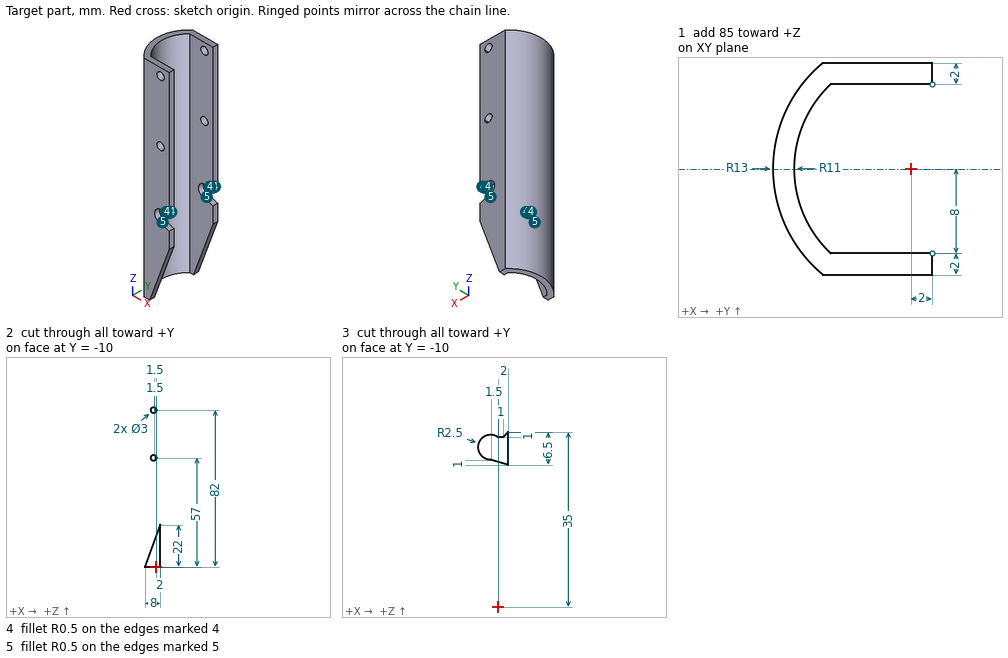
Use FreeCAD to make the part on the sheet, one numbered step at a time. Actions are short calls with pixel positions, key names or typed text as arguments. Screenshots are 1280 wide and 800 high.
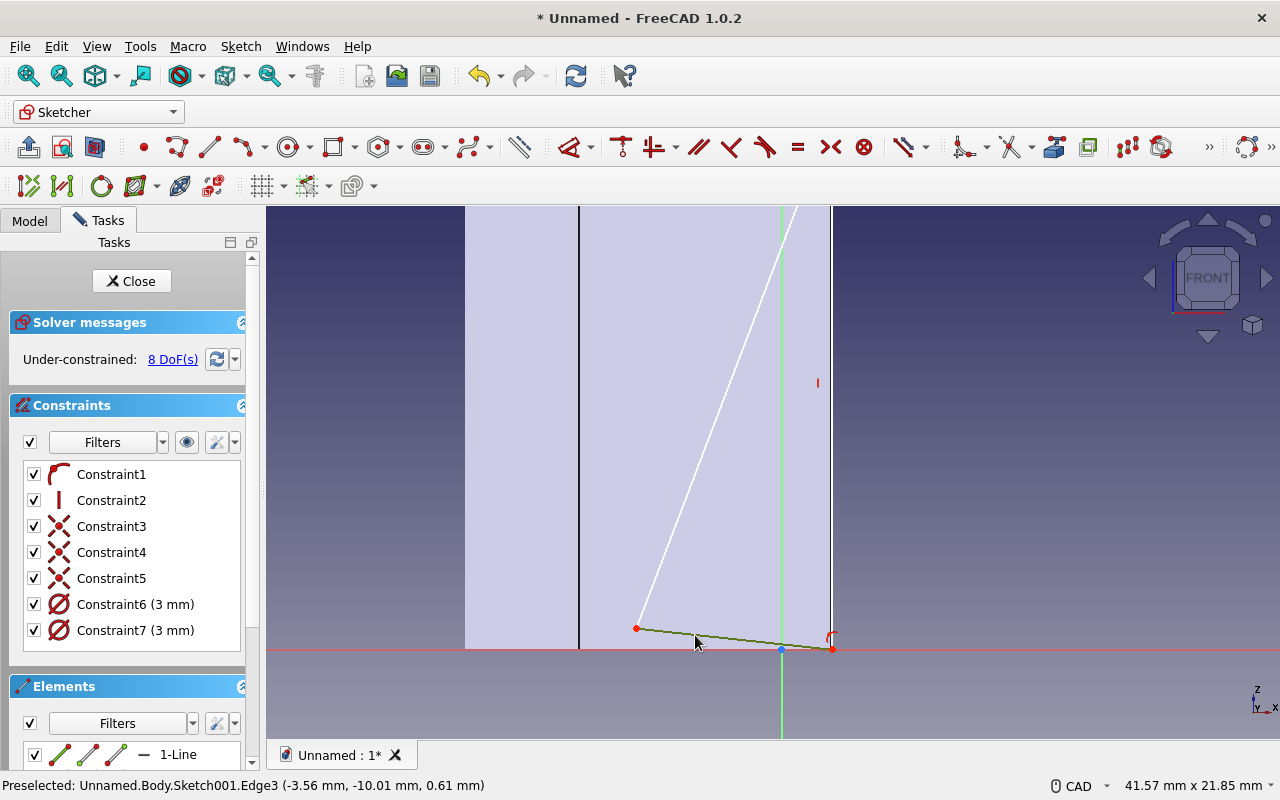
key(h)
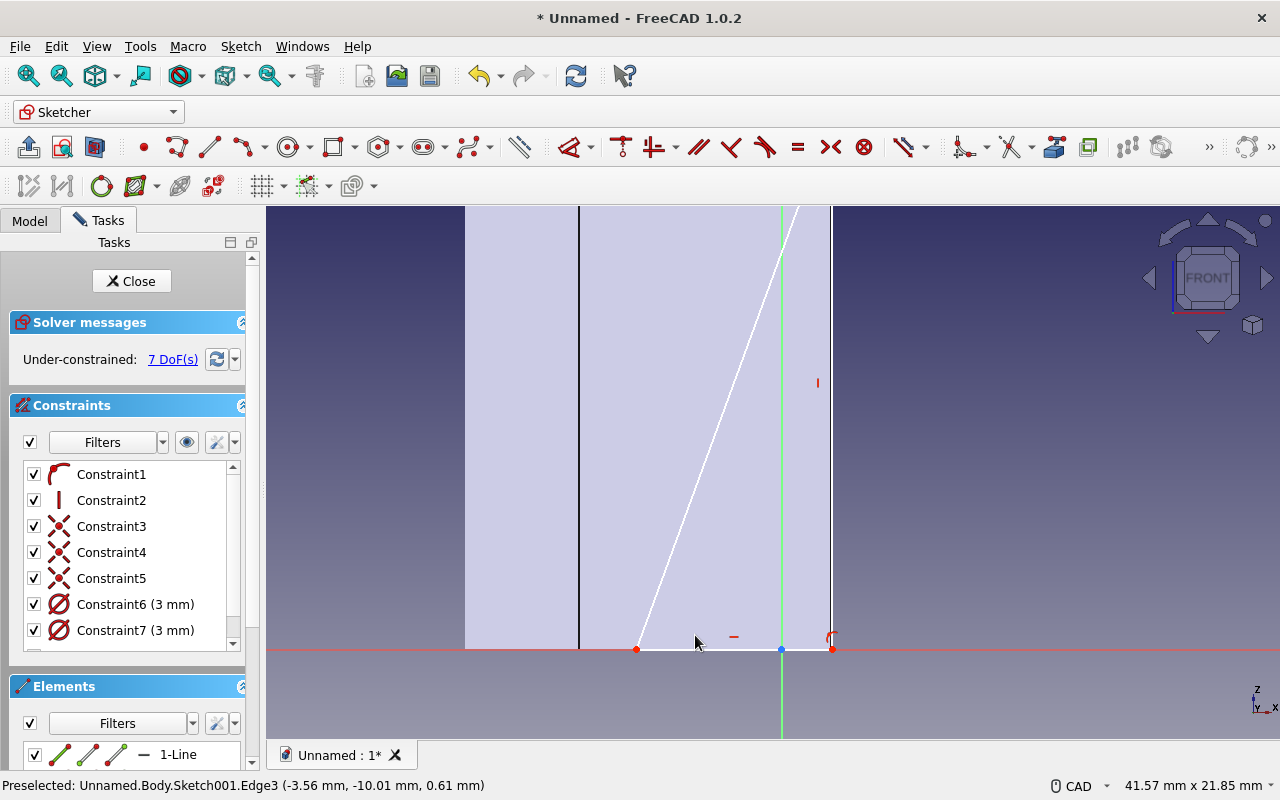
key(d)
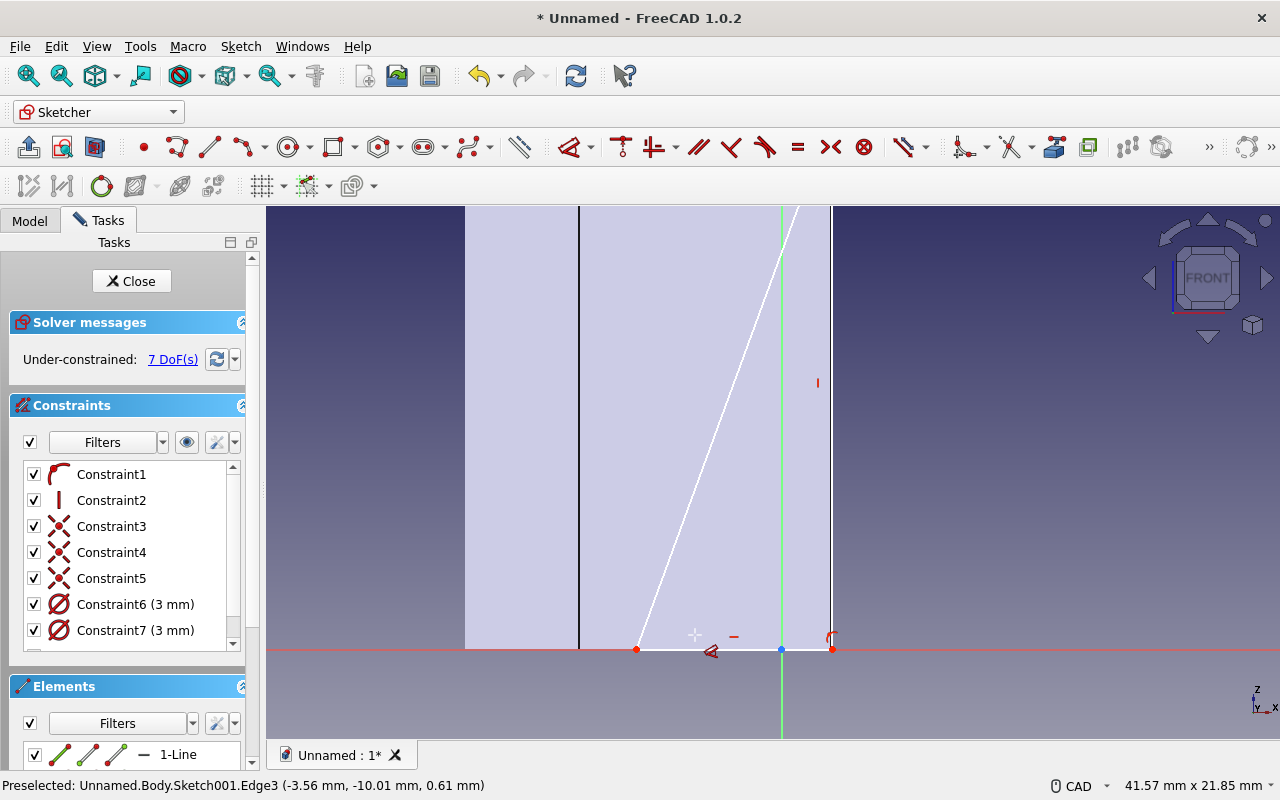
scroll(699, 639, down, 9)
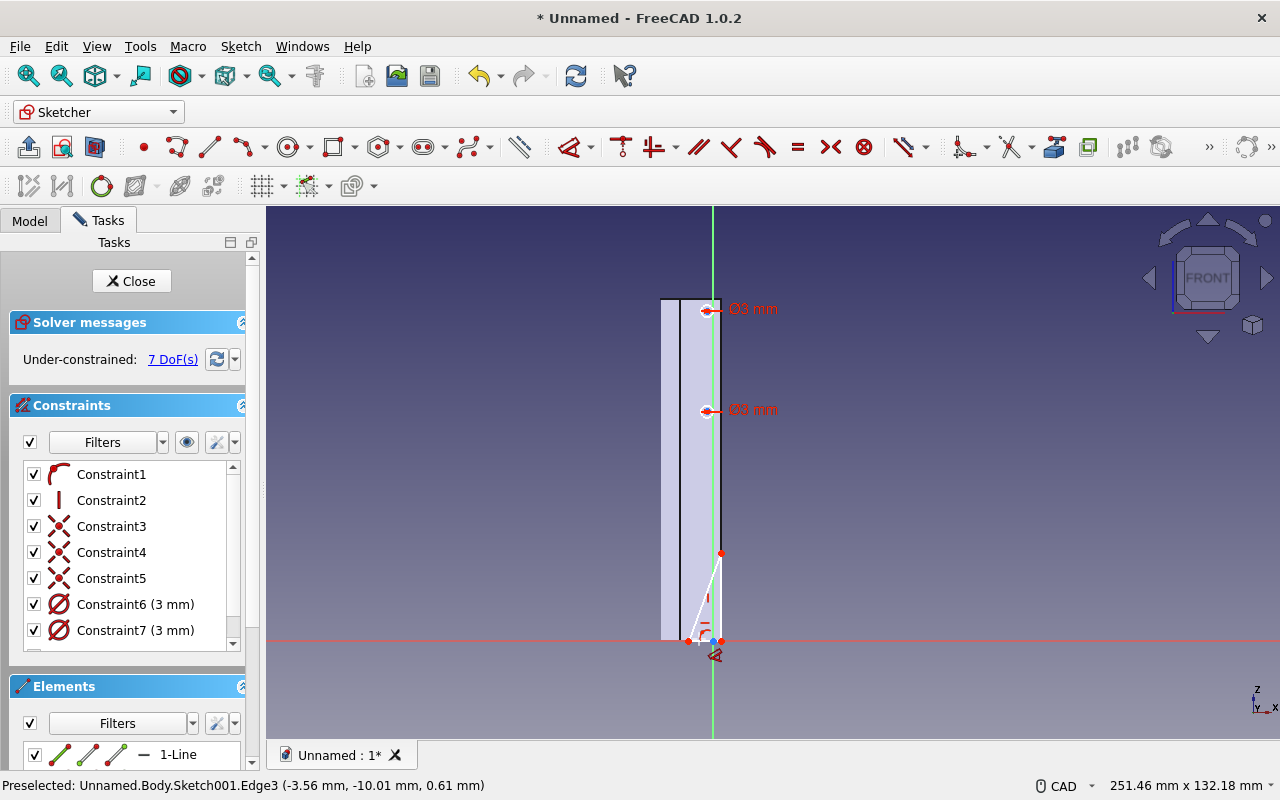
scroll(699, 641, up, 3)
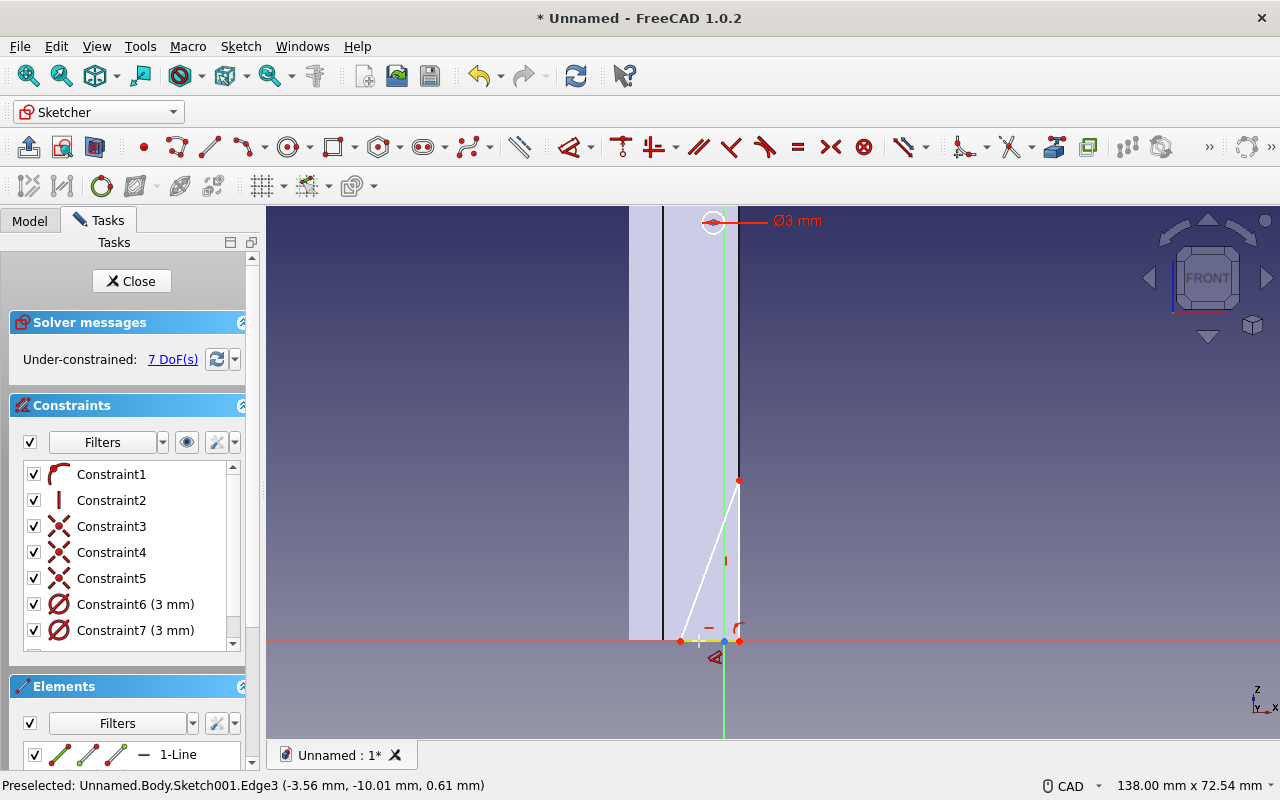
click(698, 641)
click(710, 675)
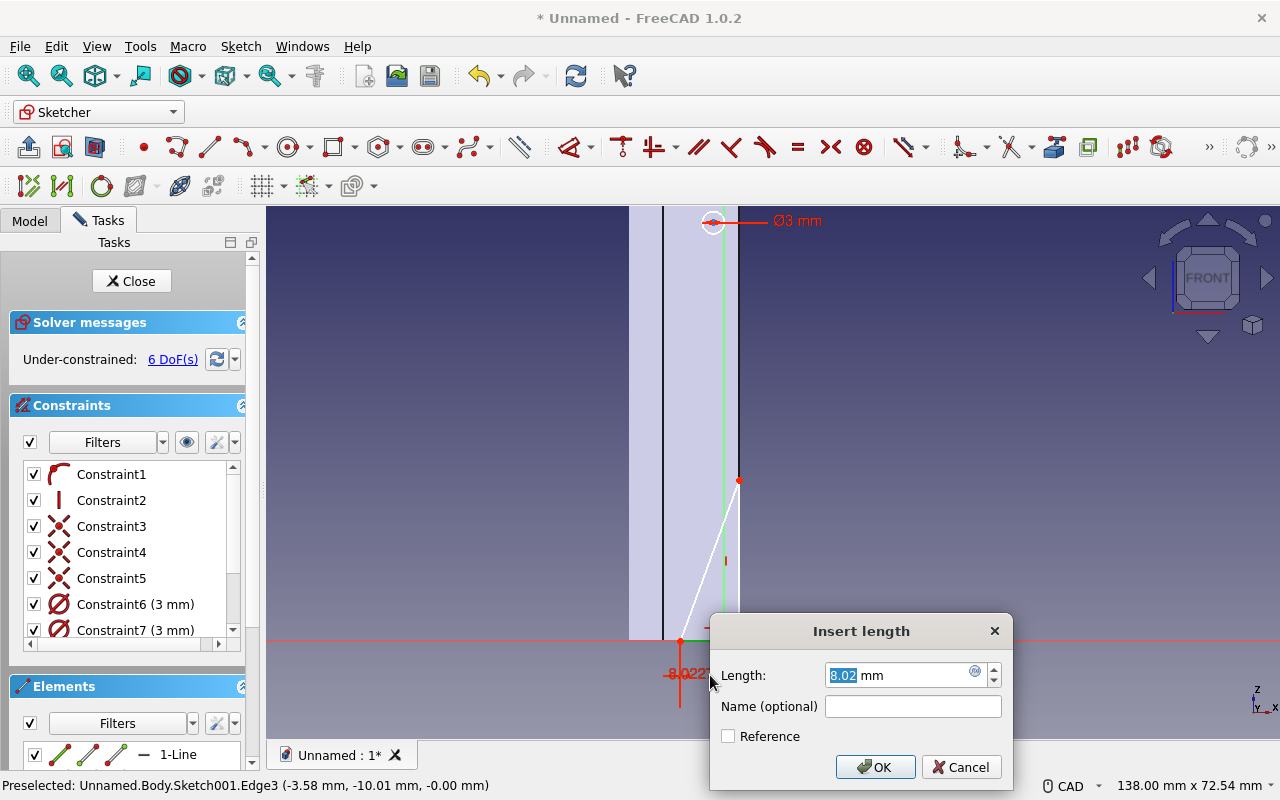
text(8)
key(Return)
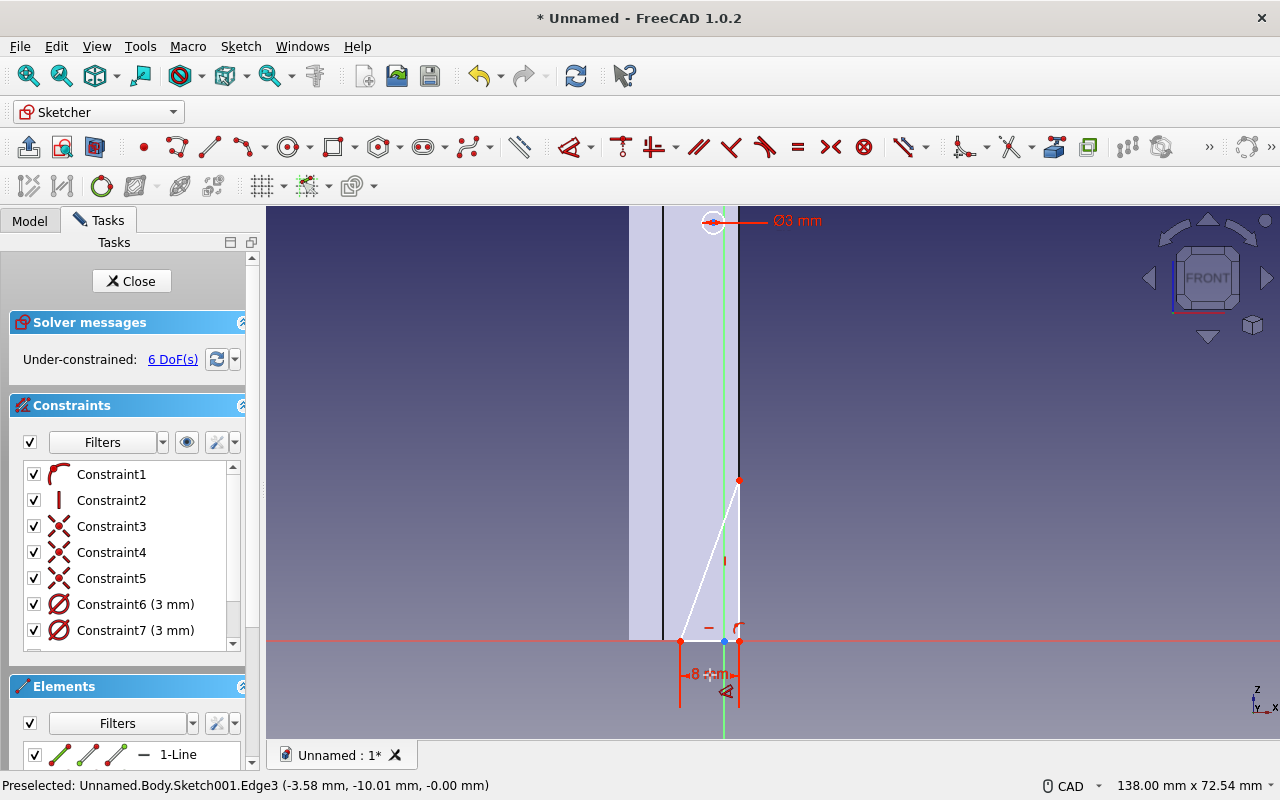
click(739, 593)
click(773, 561)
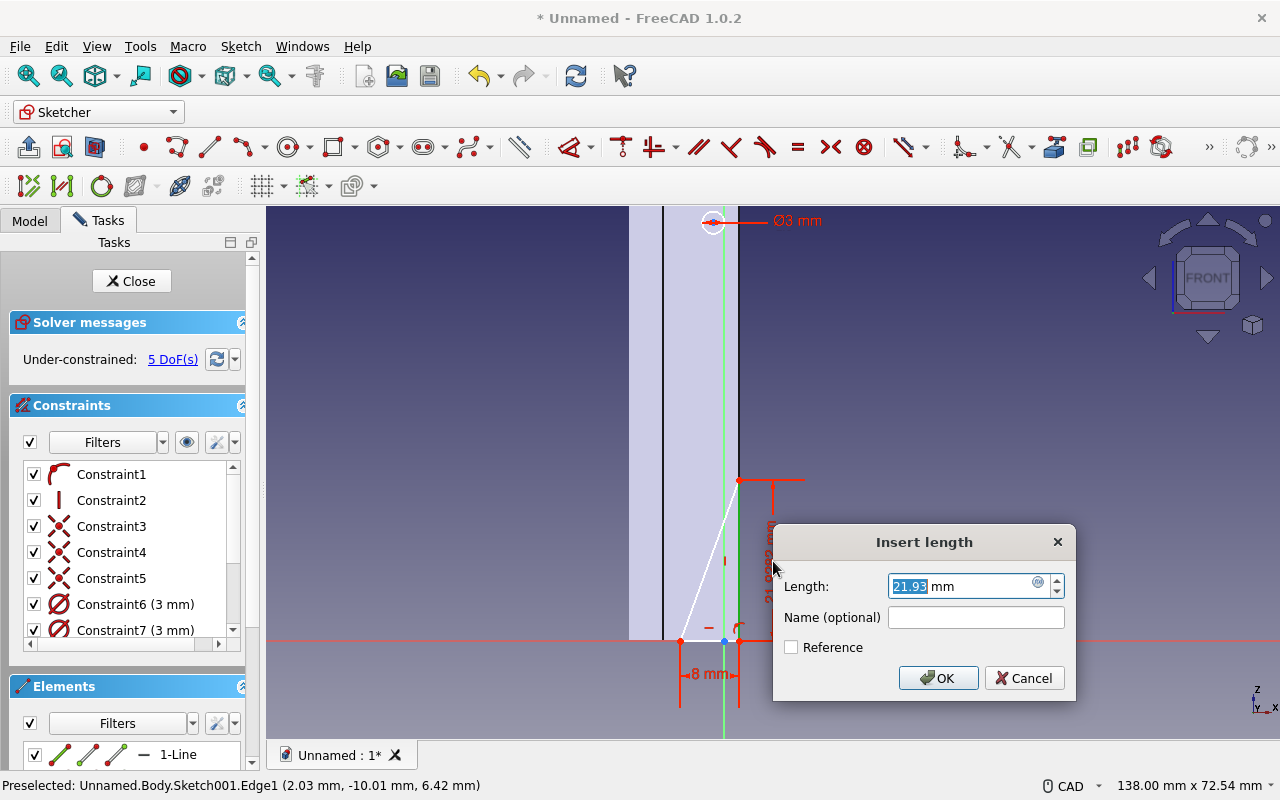
text(22)
key(Return)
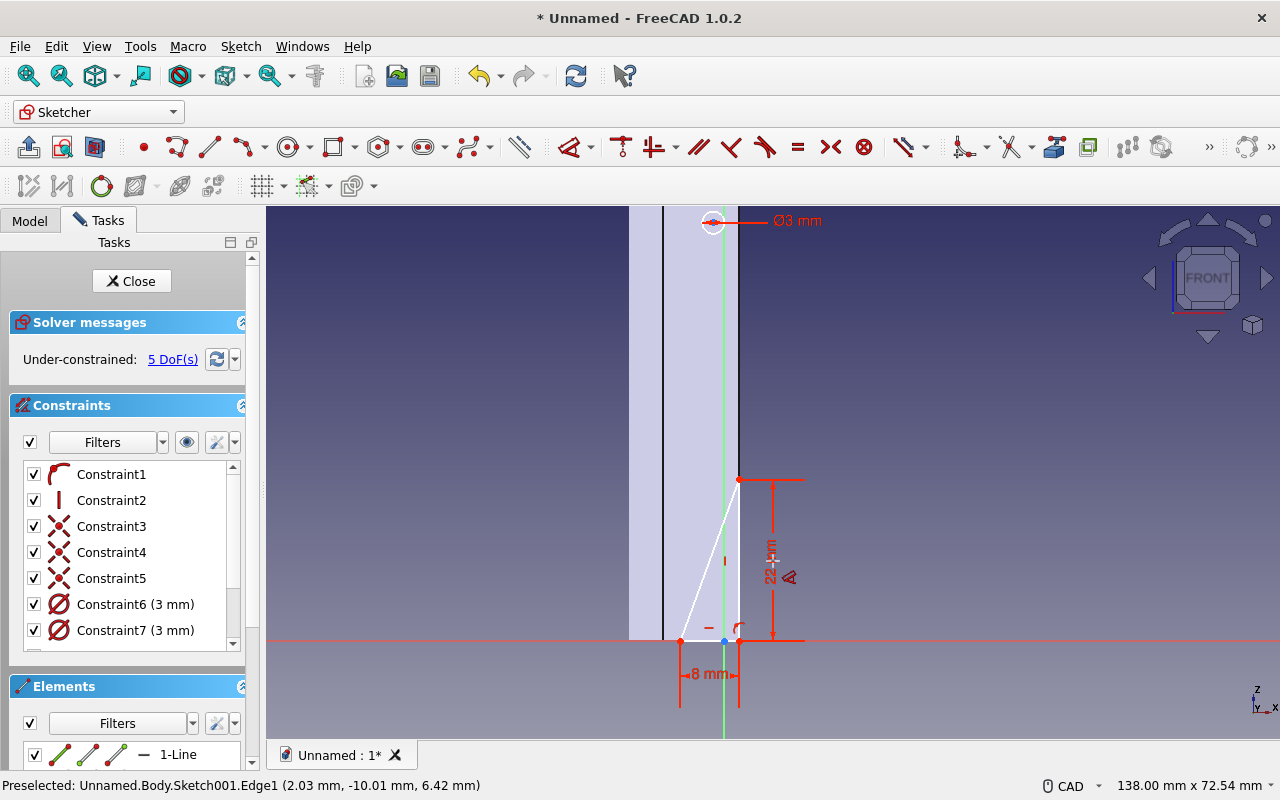
scroll(739, 641, up, 5)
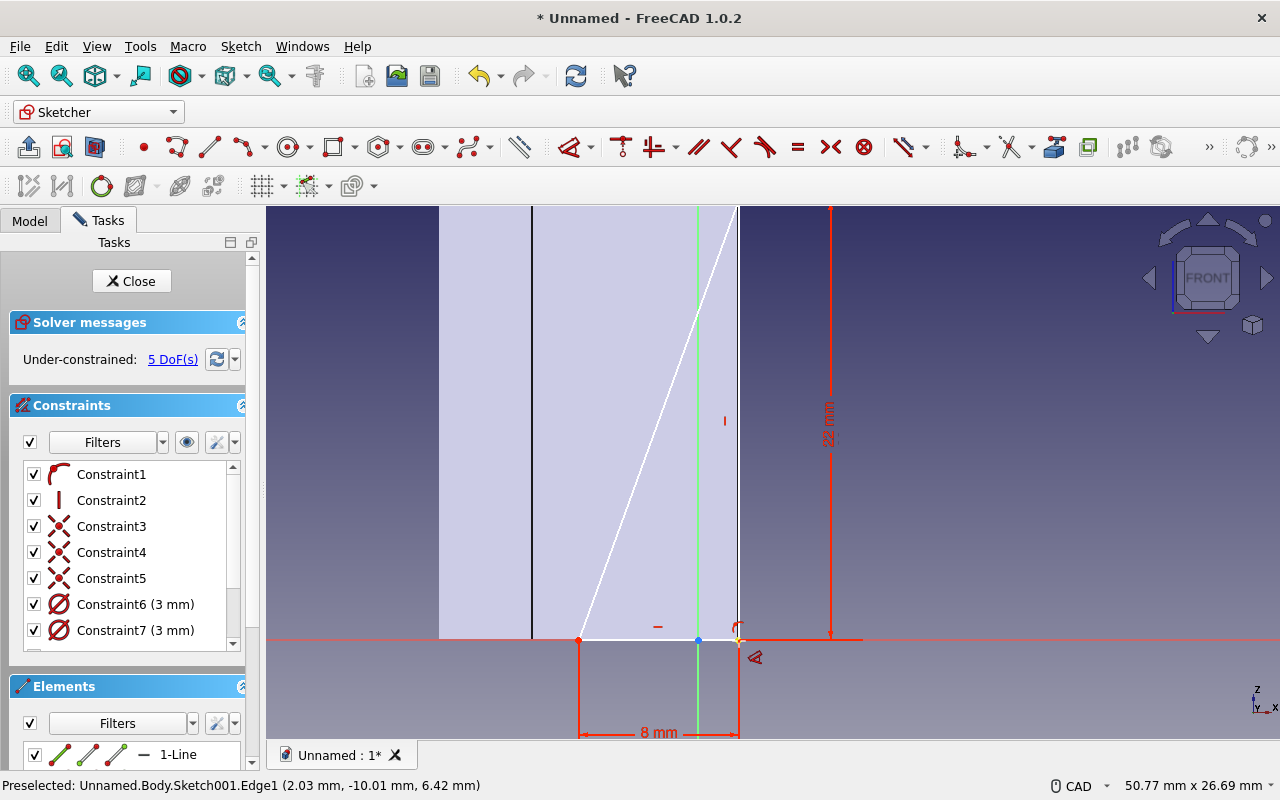
click(739, 640)
click(718, 674)